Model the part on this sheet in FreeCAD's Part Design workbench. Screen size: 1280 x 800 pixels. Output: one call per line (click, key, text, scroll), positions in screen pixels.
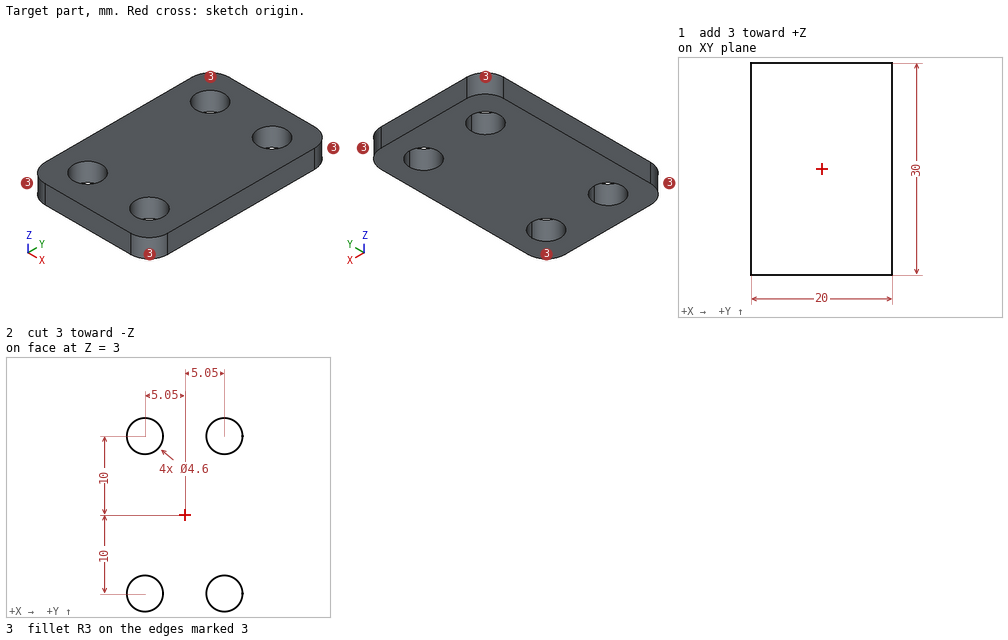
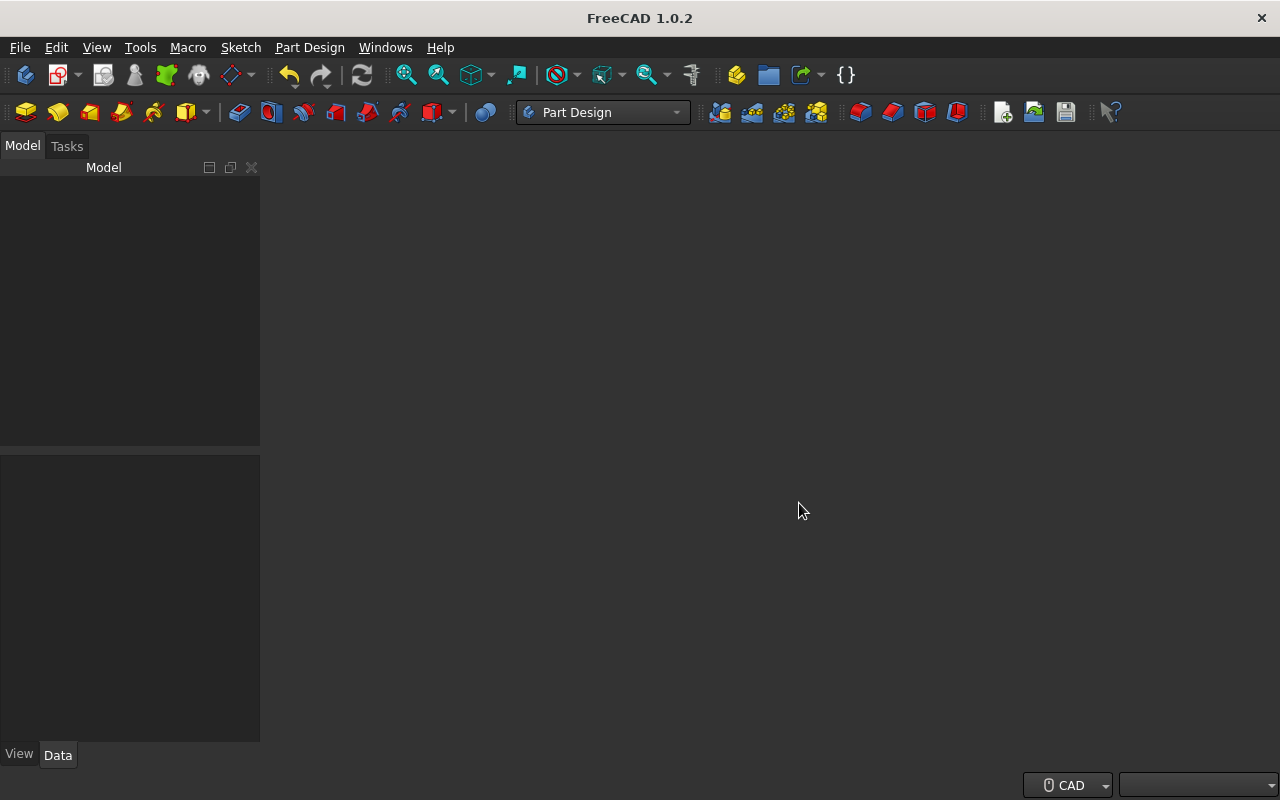
click(1002, 112)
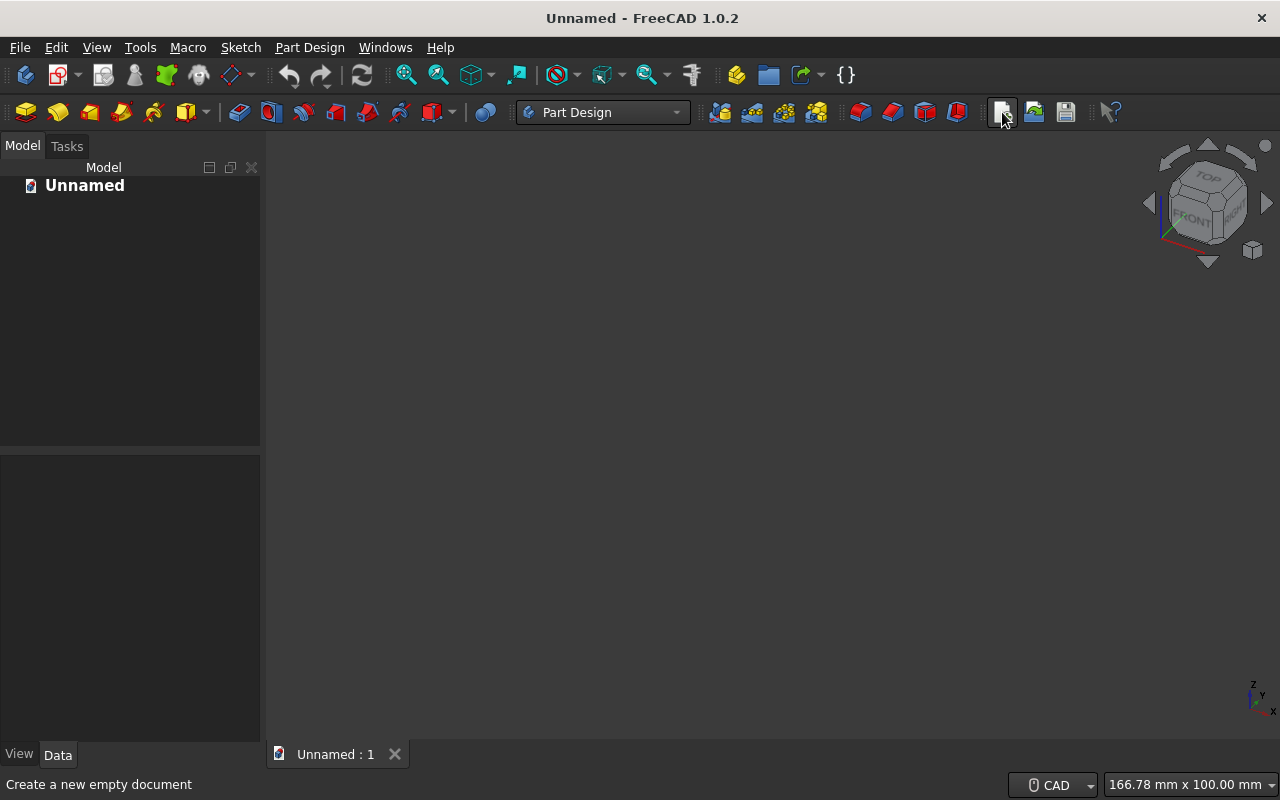
click(58, 76)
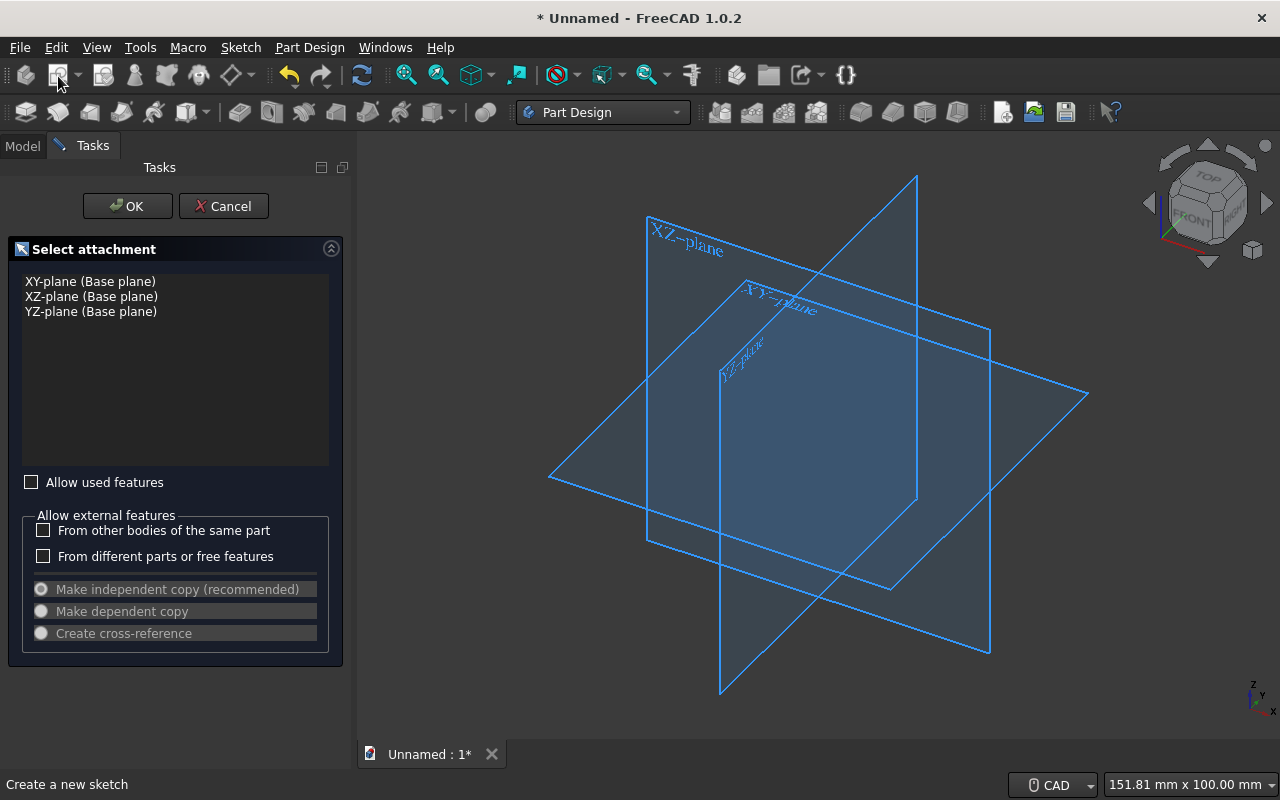
click(82, 282)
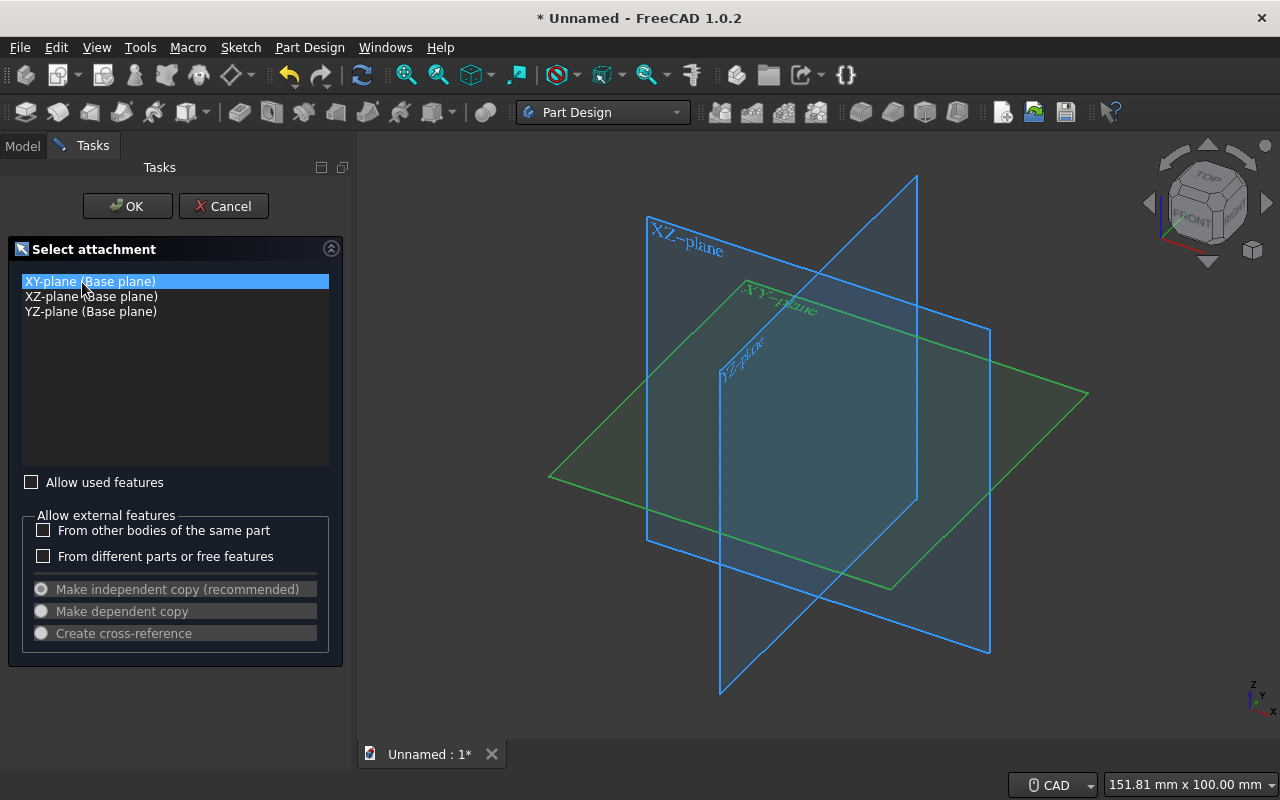
click(128, 206)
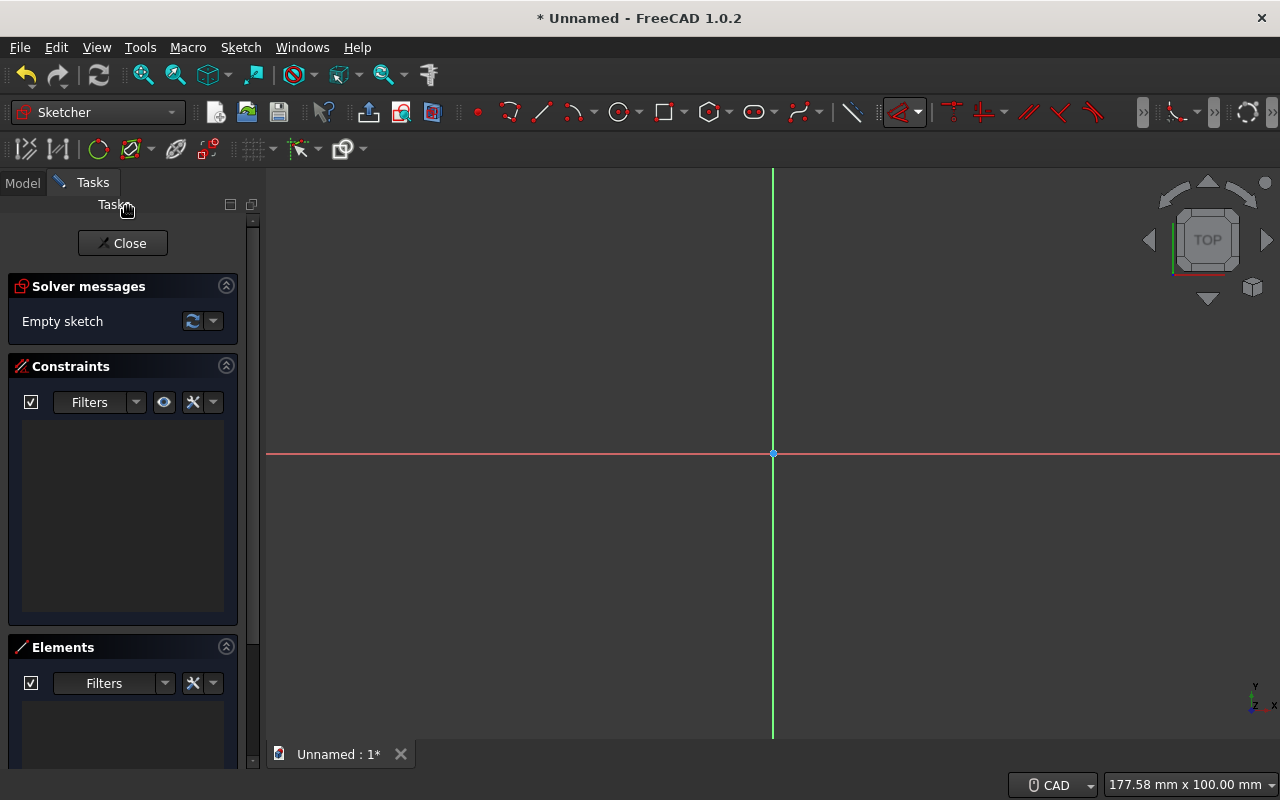
scroll(829, 454, up, 4)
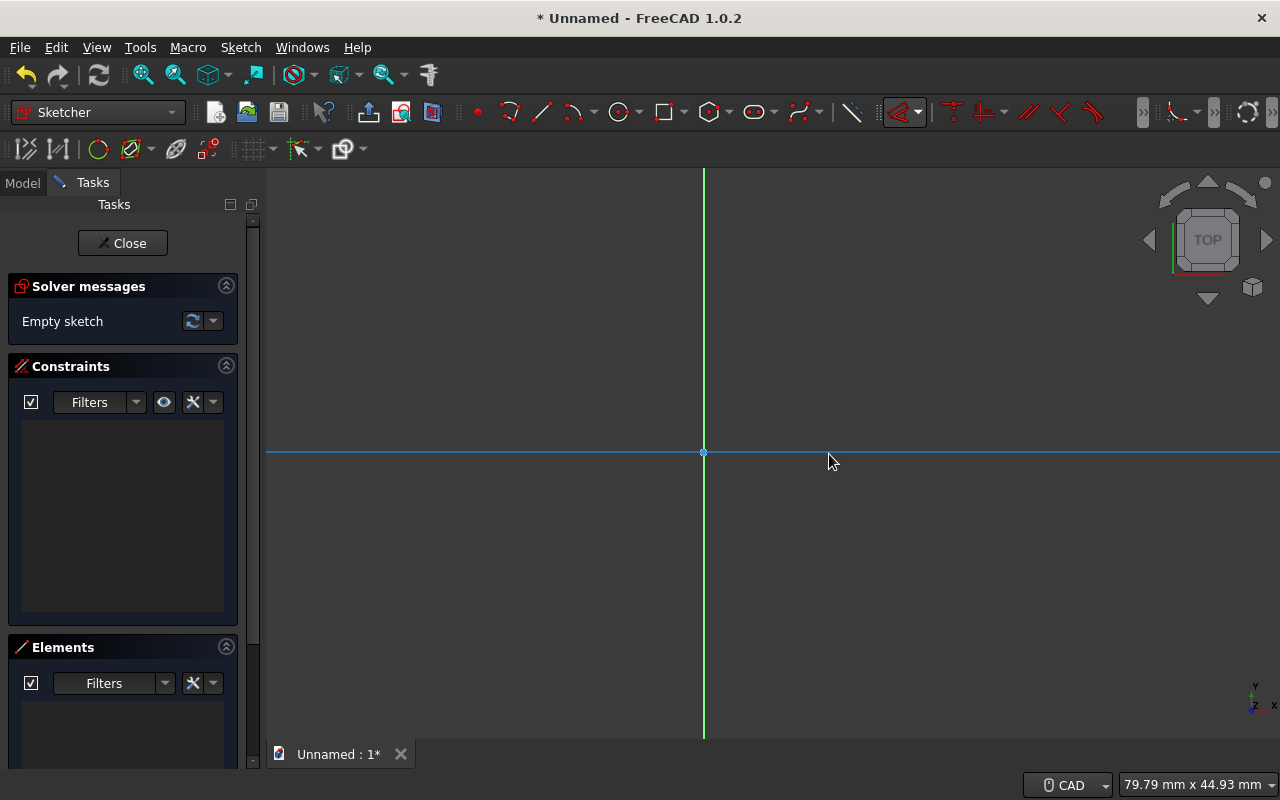
key(g)
key(v)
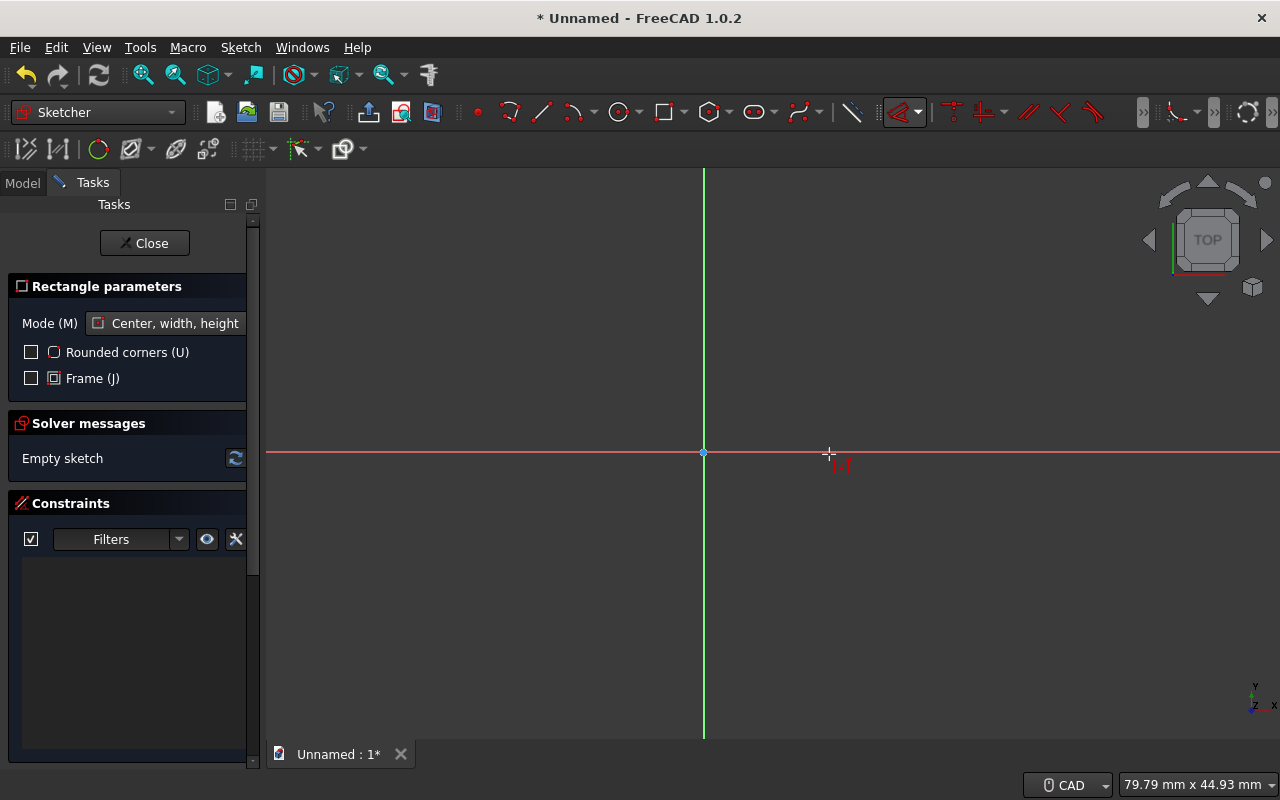
click(704, 452)
click(831, 262)
key(Escape)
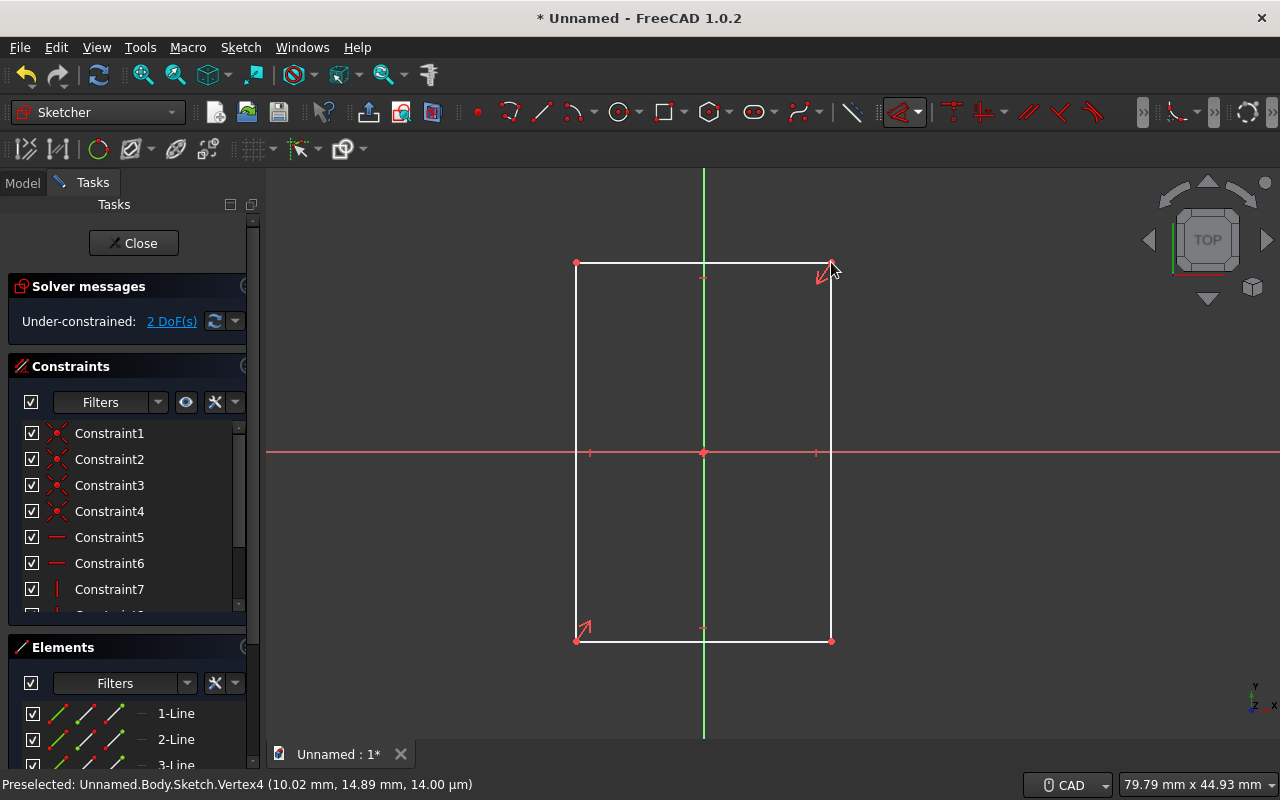
click(898, 112)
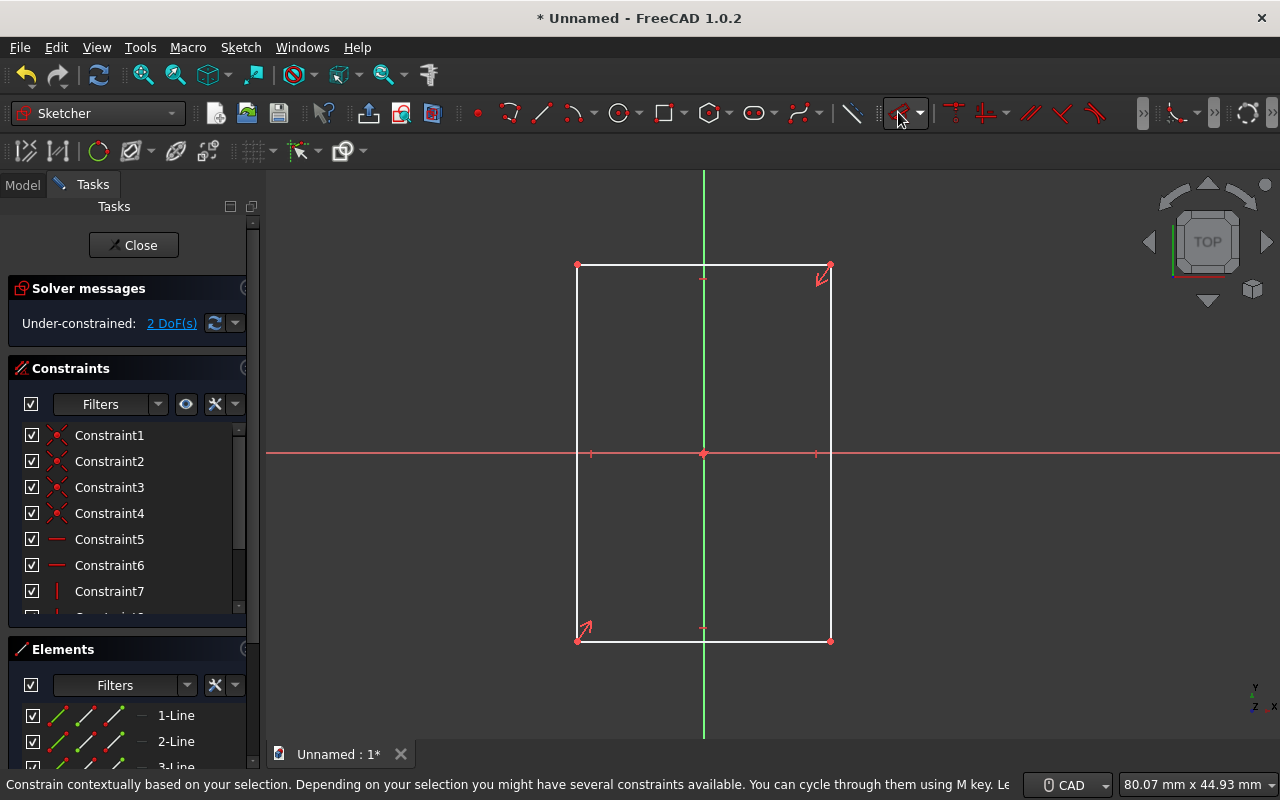
click(653, 642)
click(646, 676)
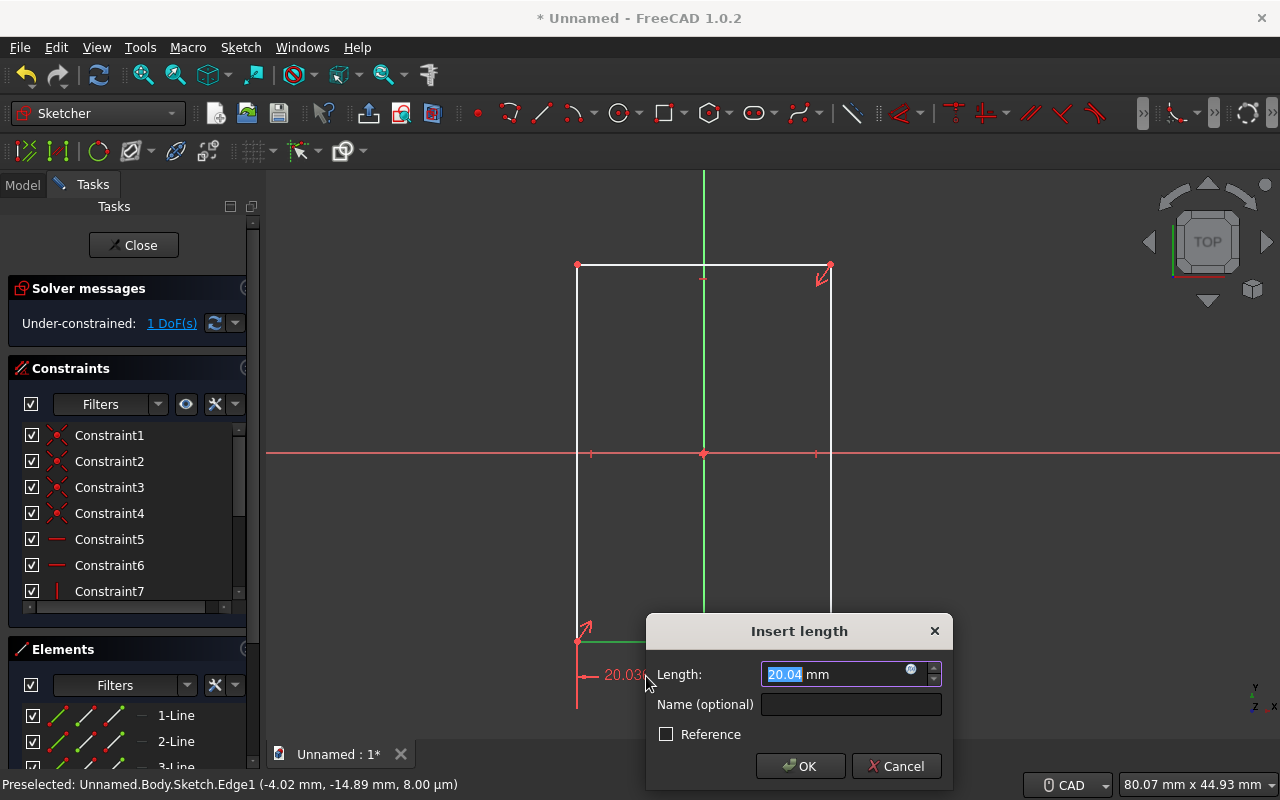
text(20)
key(Return)